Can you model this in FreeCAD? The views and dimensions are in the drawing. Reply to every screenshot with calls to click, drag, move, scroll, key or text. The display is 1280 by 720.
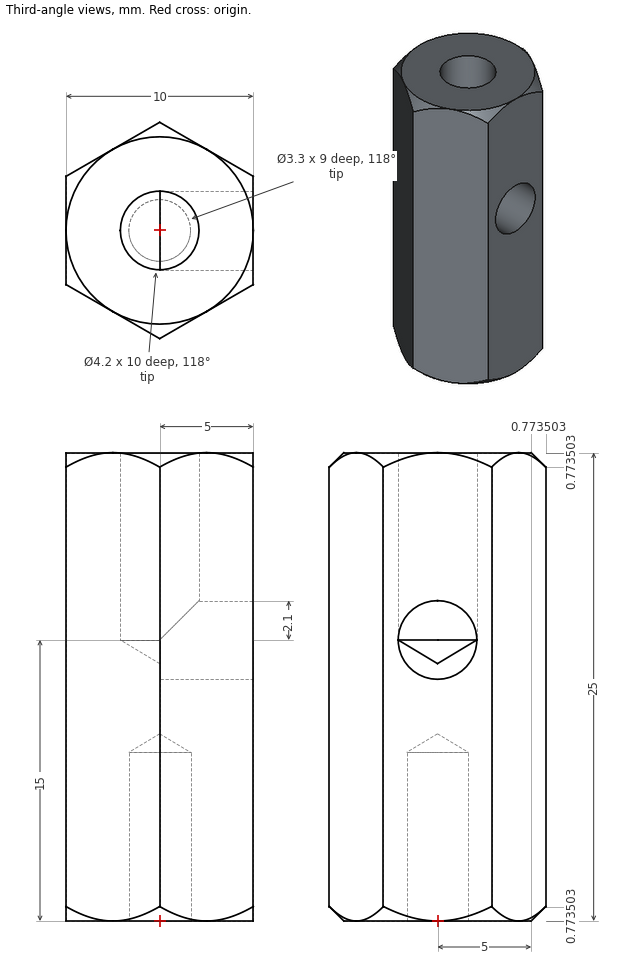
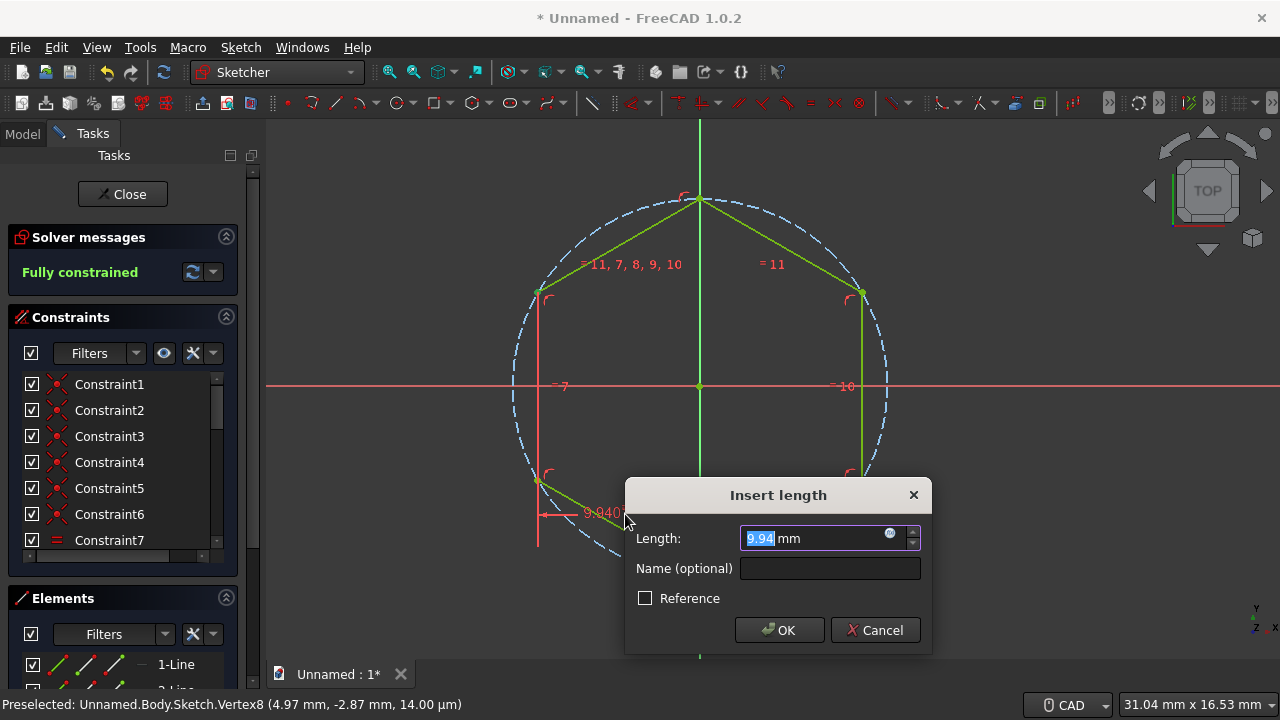
text(10)
key(Return)
key(Escape)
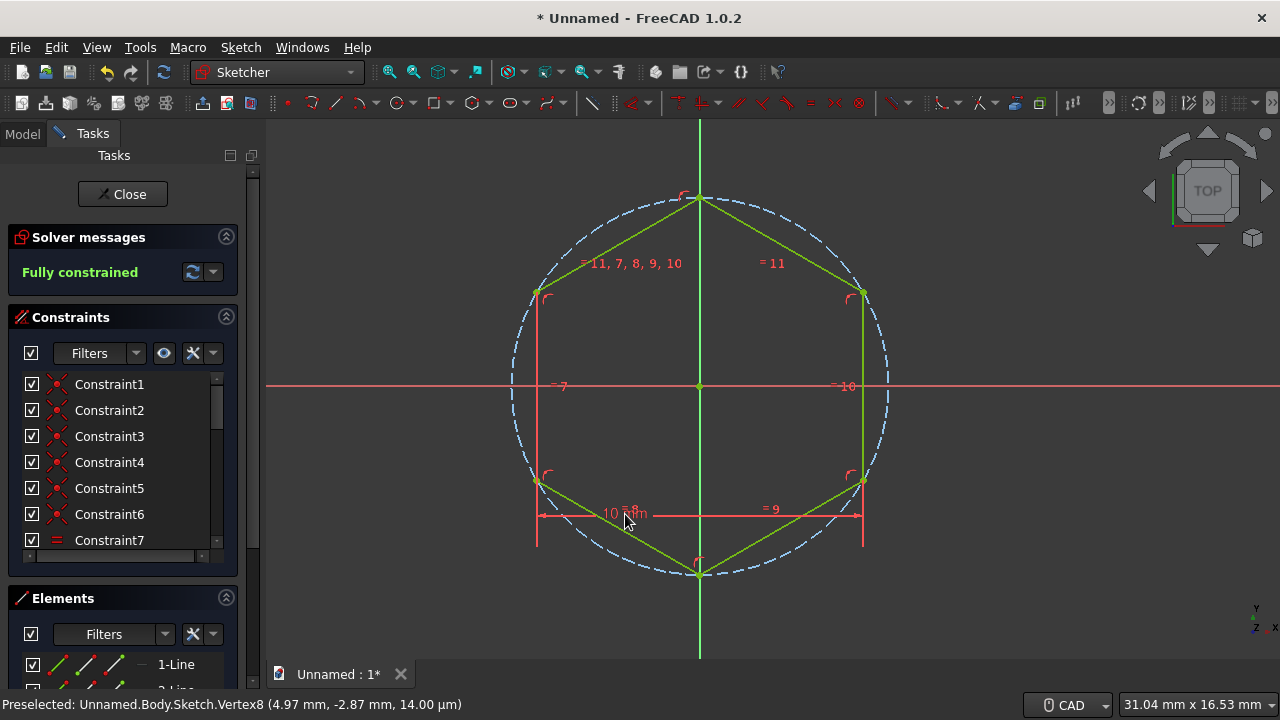
click(123, 194)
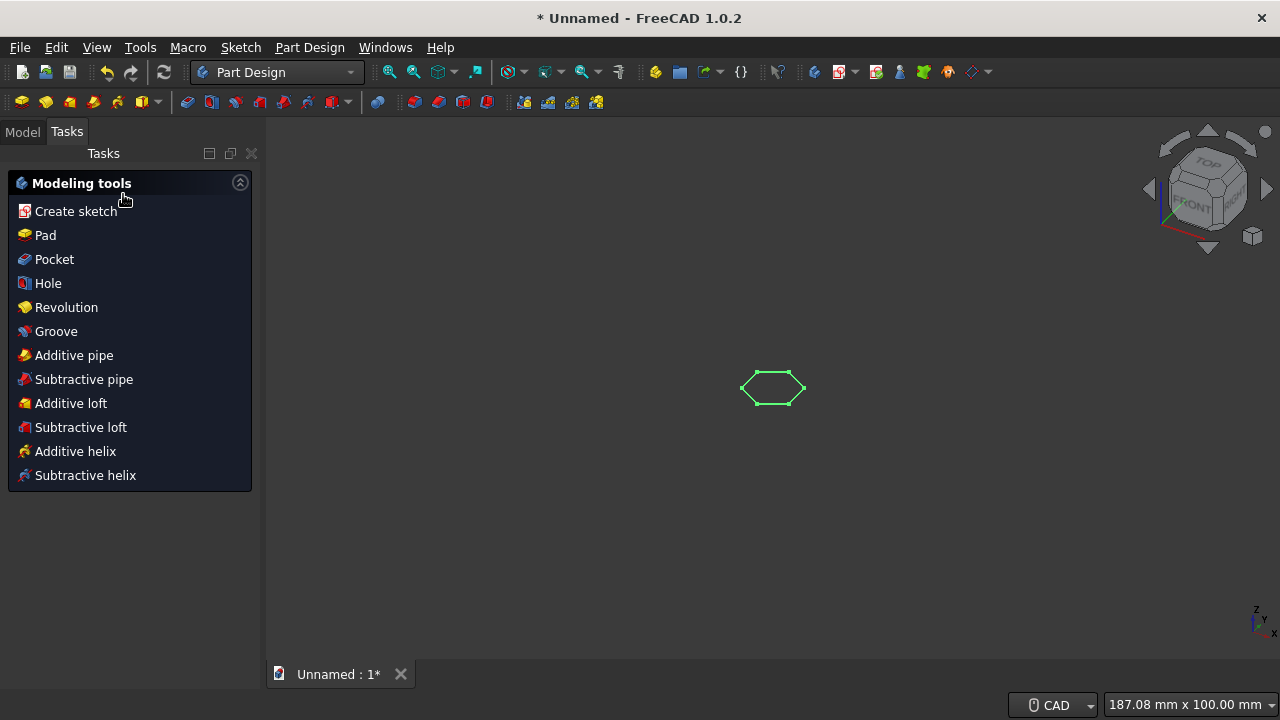
click(22, 102)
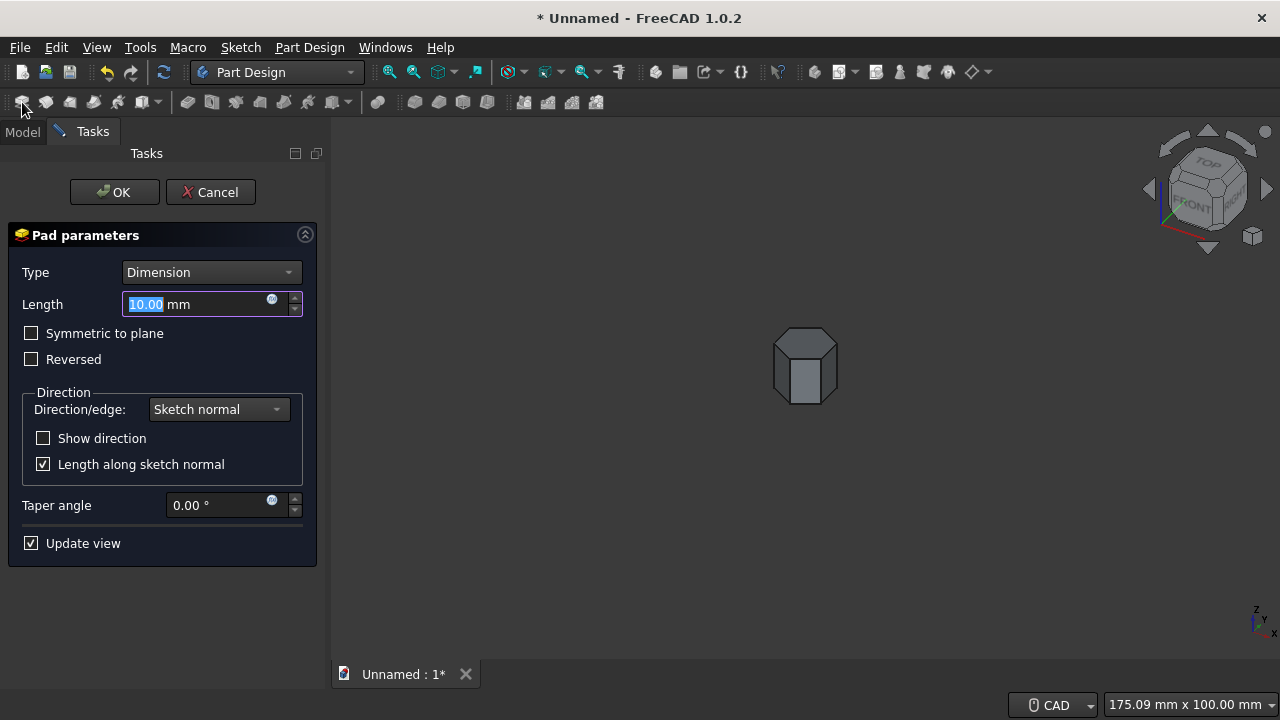
text(25)
key(Tab)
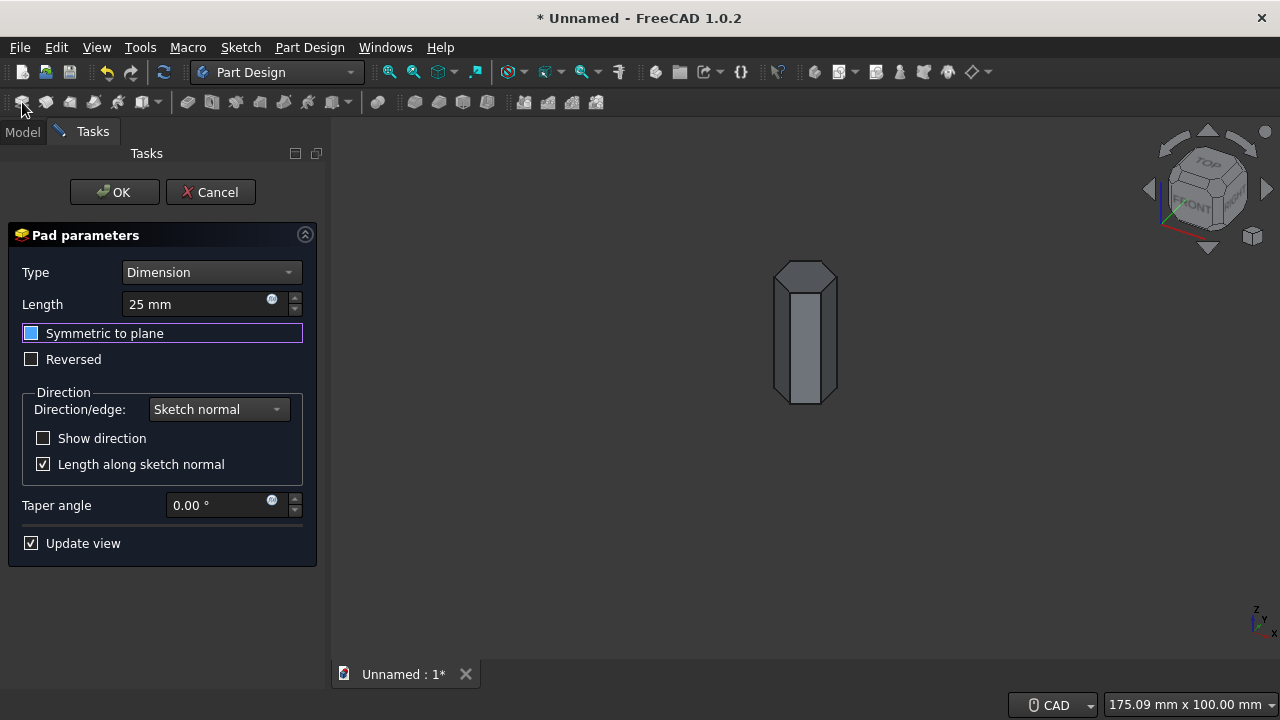
click(115, 192)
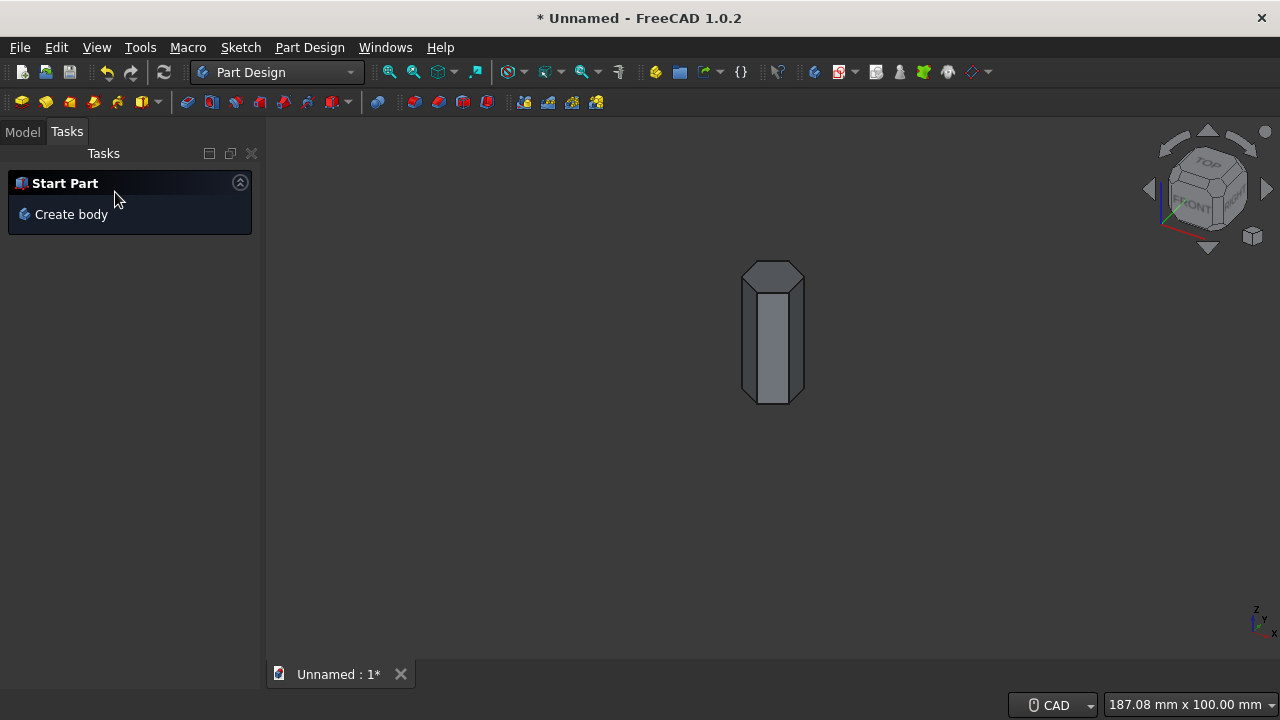
key(v)
key(f)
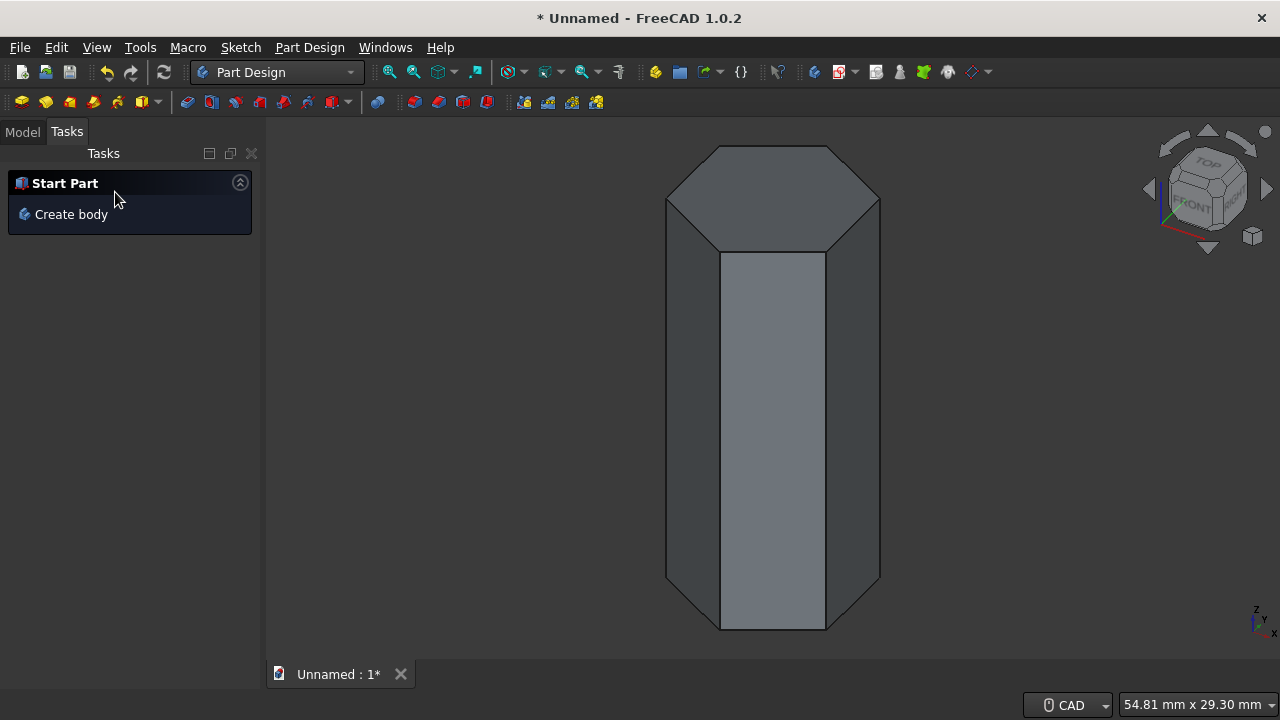
click(773, 198)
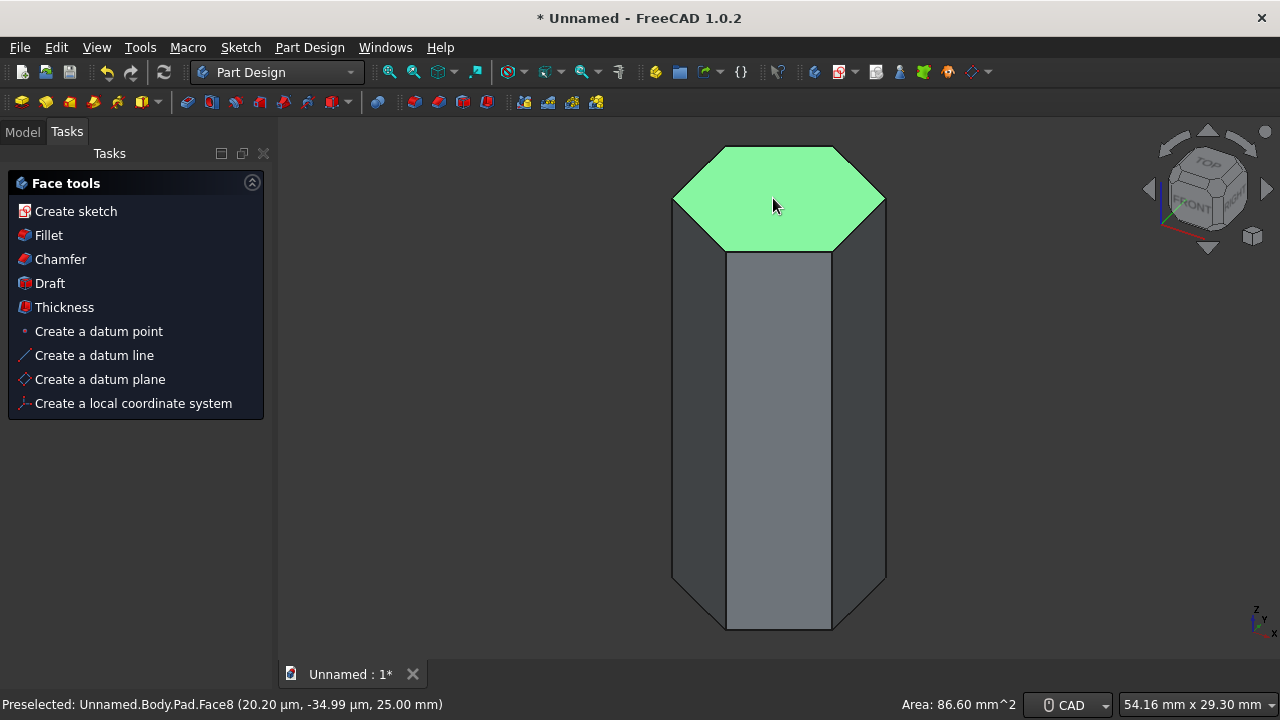
click(840, 72)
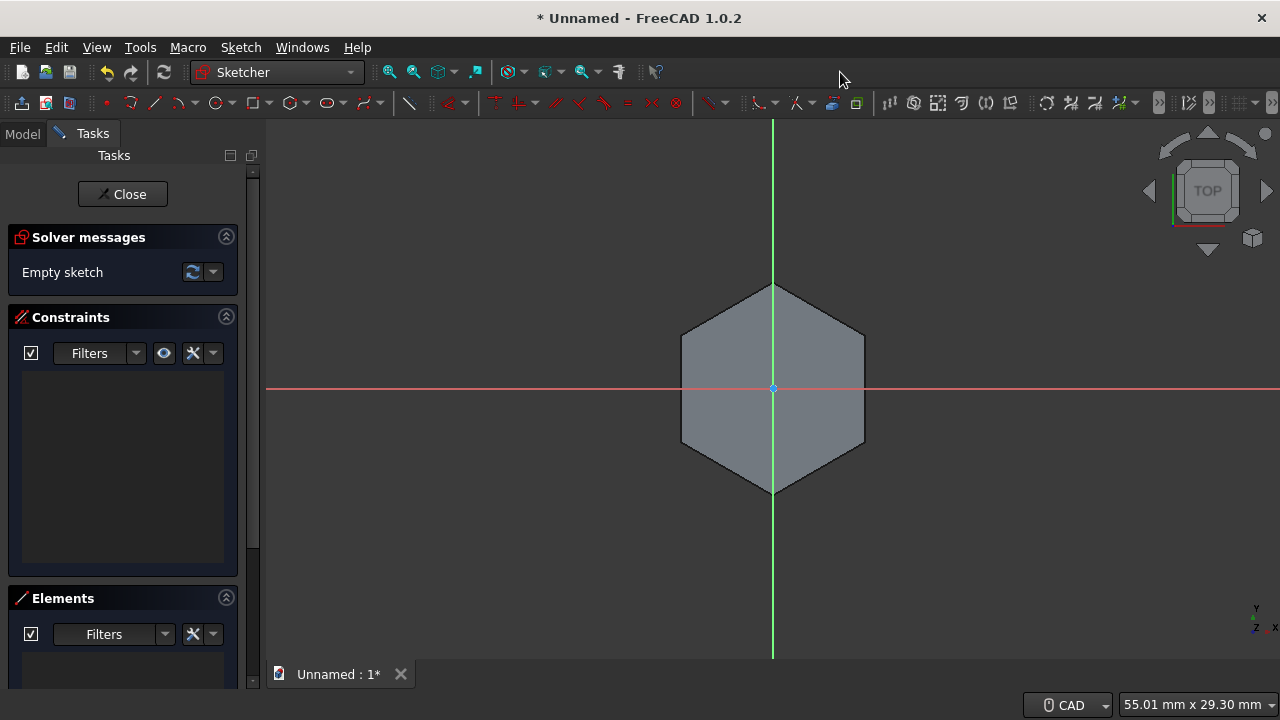
scroll(795, 389, up, 7)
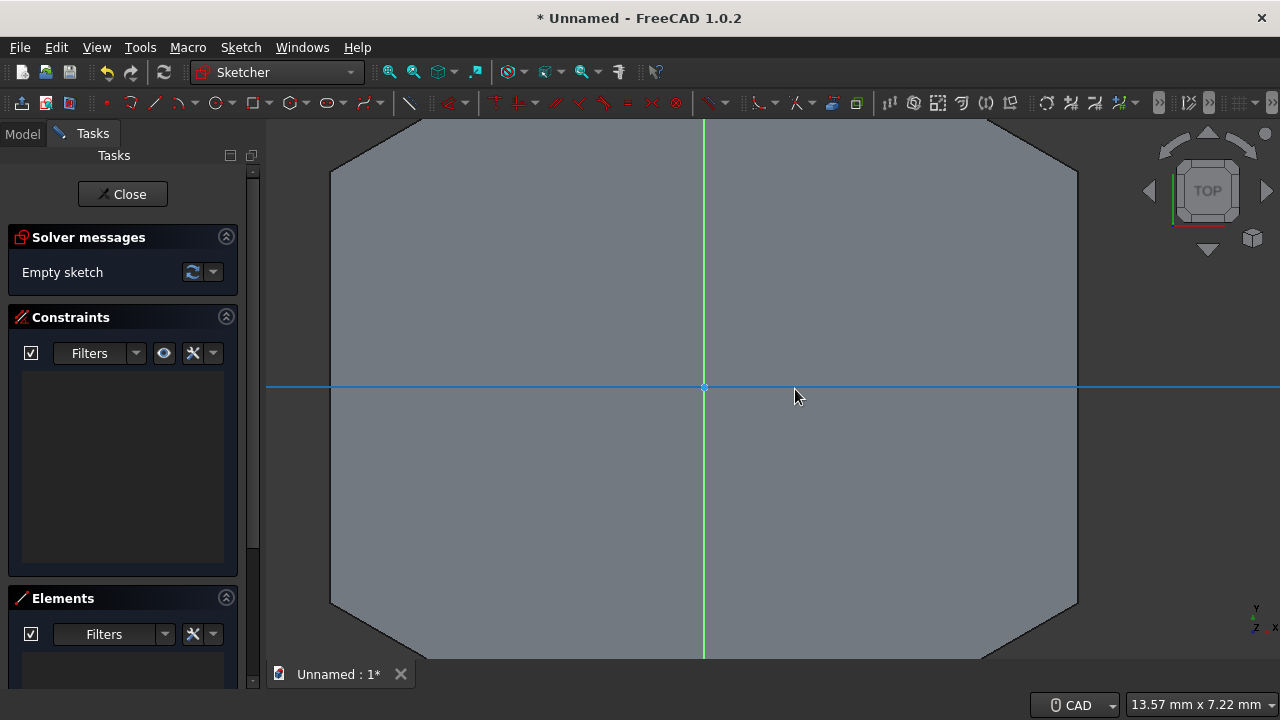
click(216, 104)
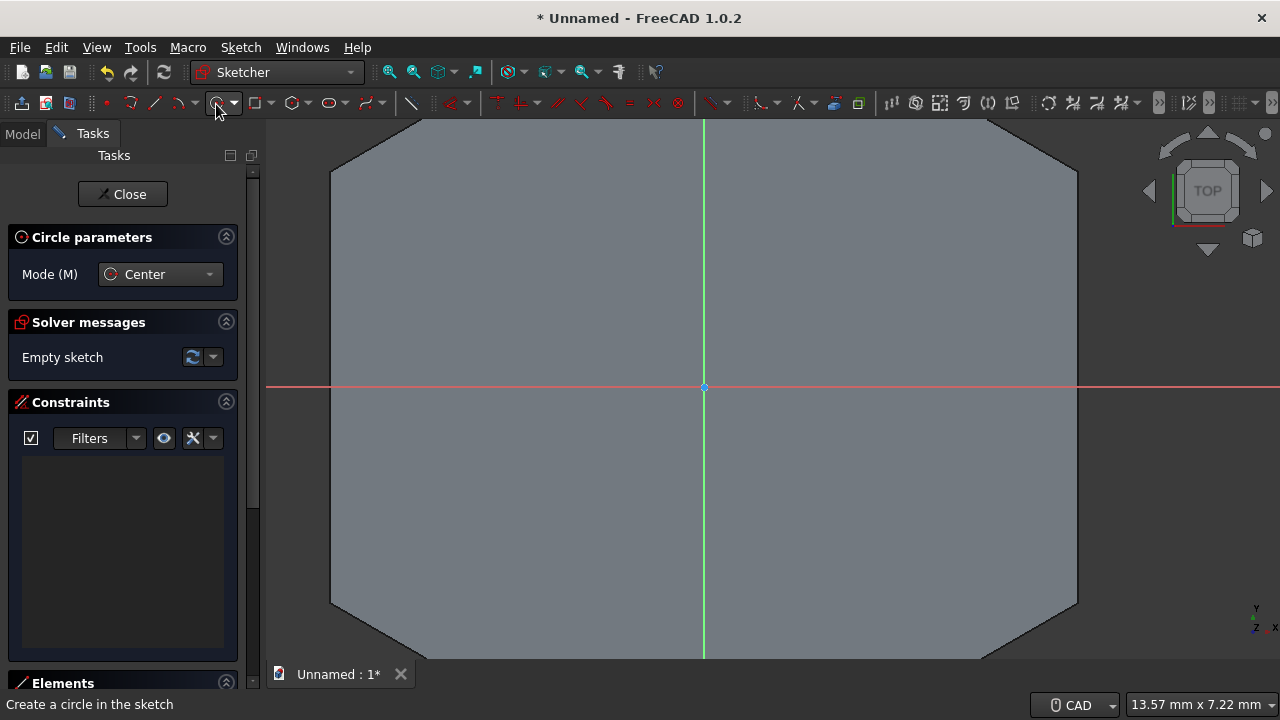
click(704, 387)
move(815, 276)